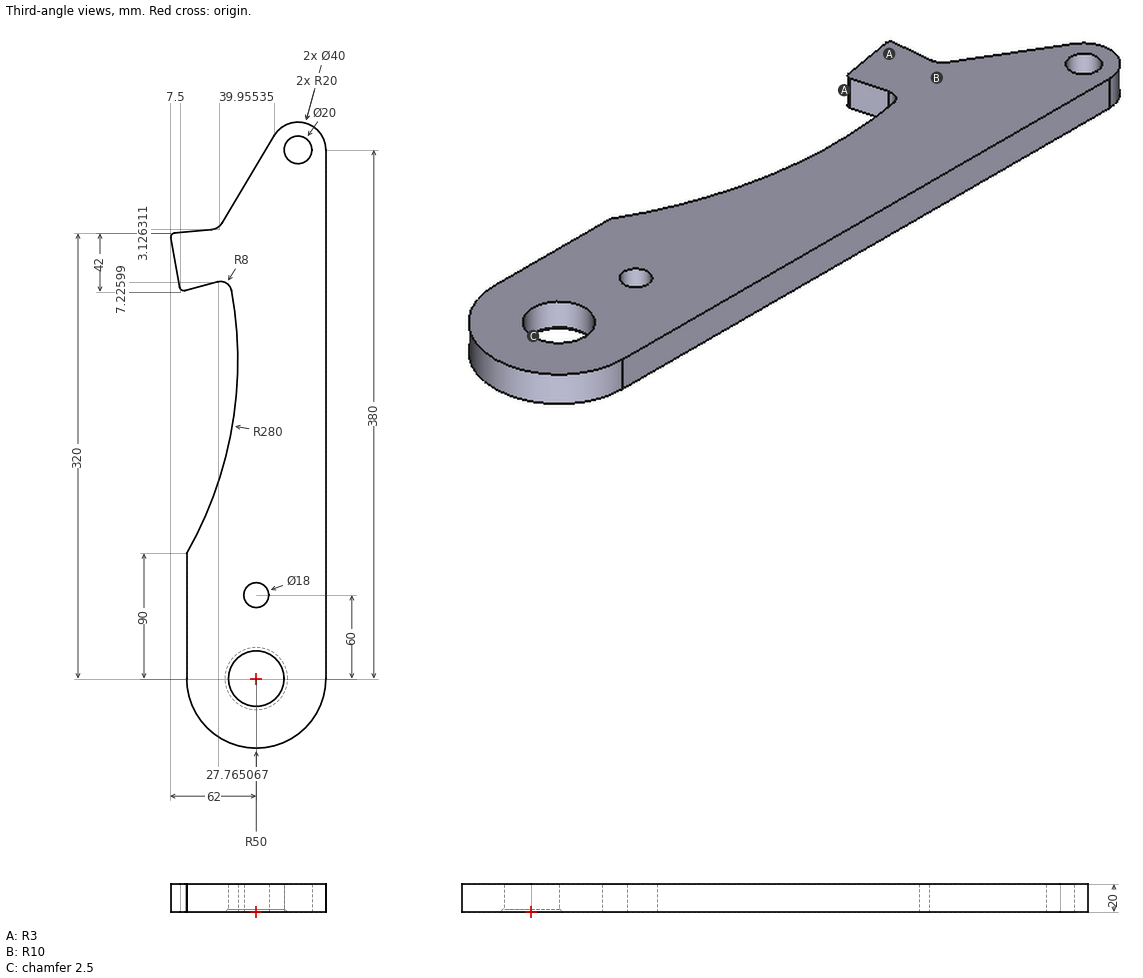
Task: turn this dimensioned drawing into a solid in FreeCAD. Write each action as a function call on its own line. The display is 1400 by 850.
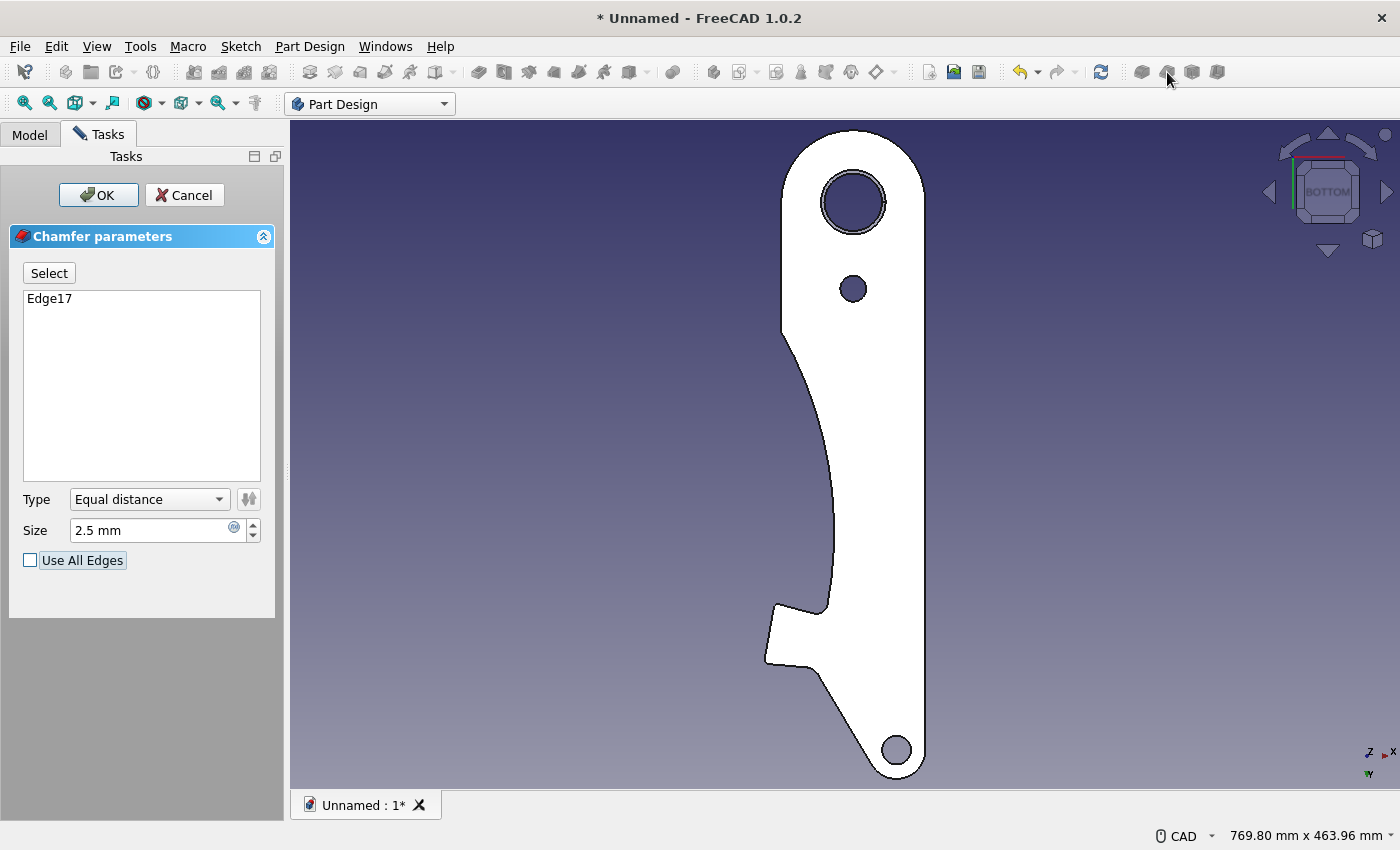
click(99, 195)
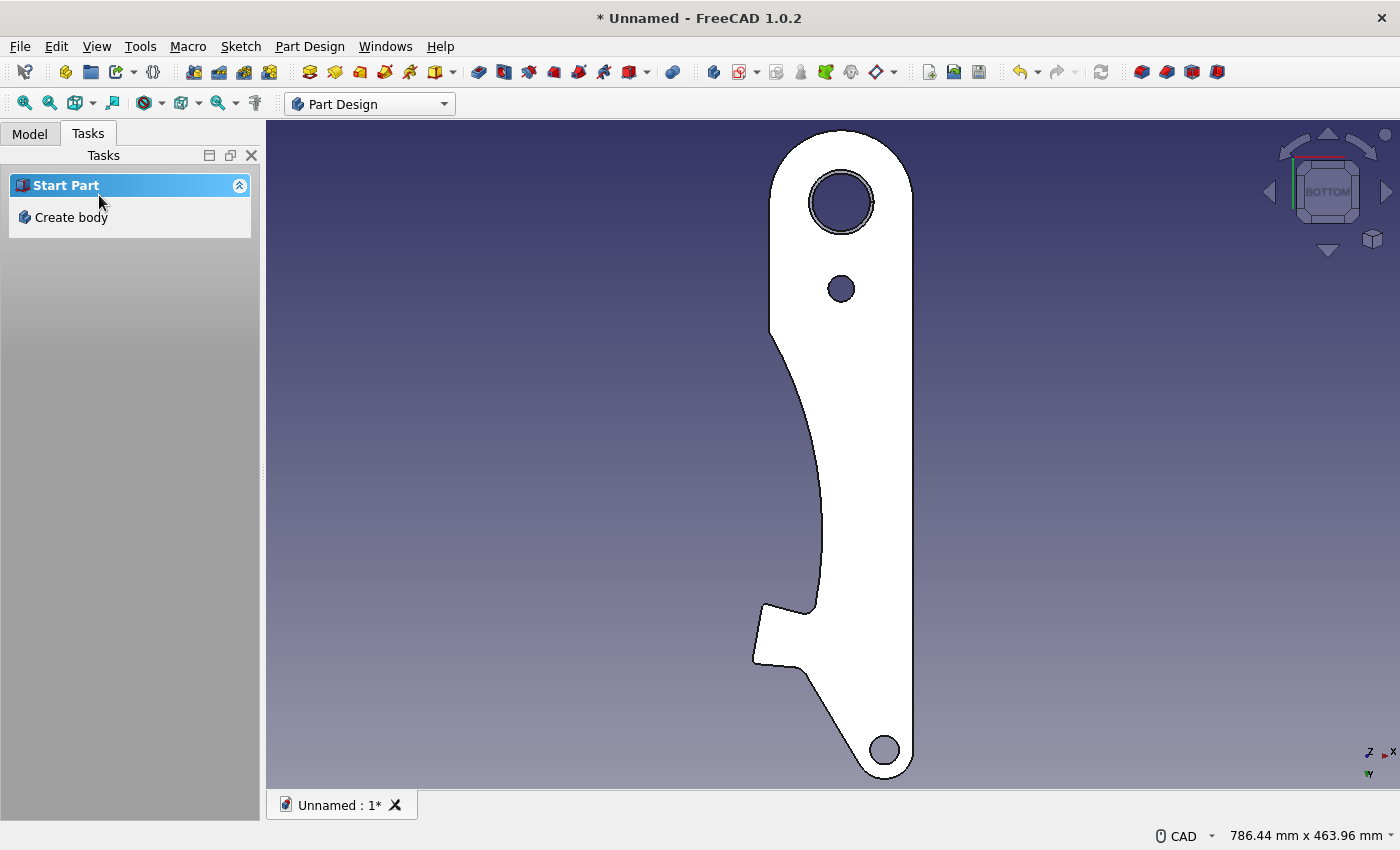
key(0)